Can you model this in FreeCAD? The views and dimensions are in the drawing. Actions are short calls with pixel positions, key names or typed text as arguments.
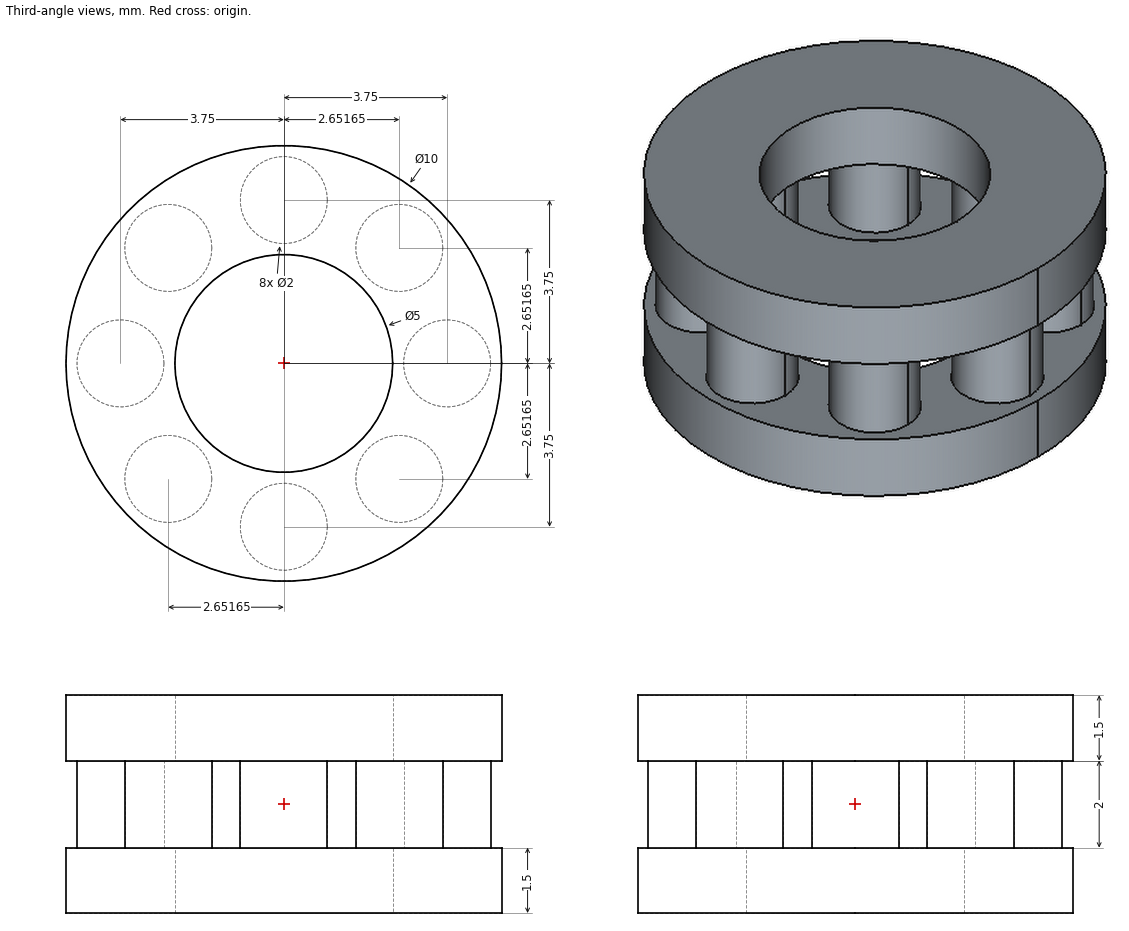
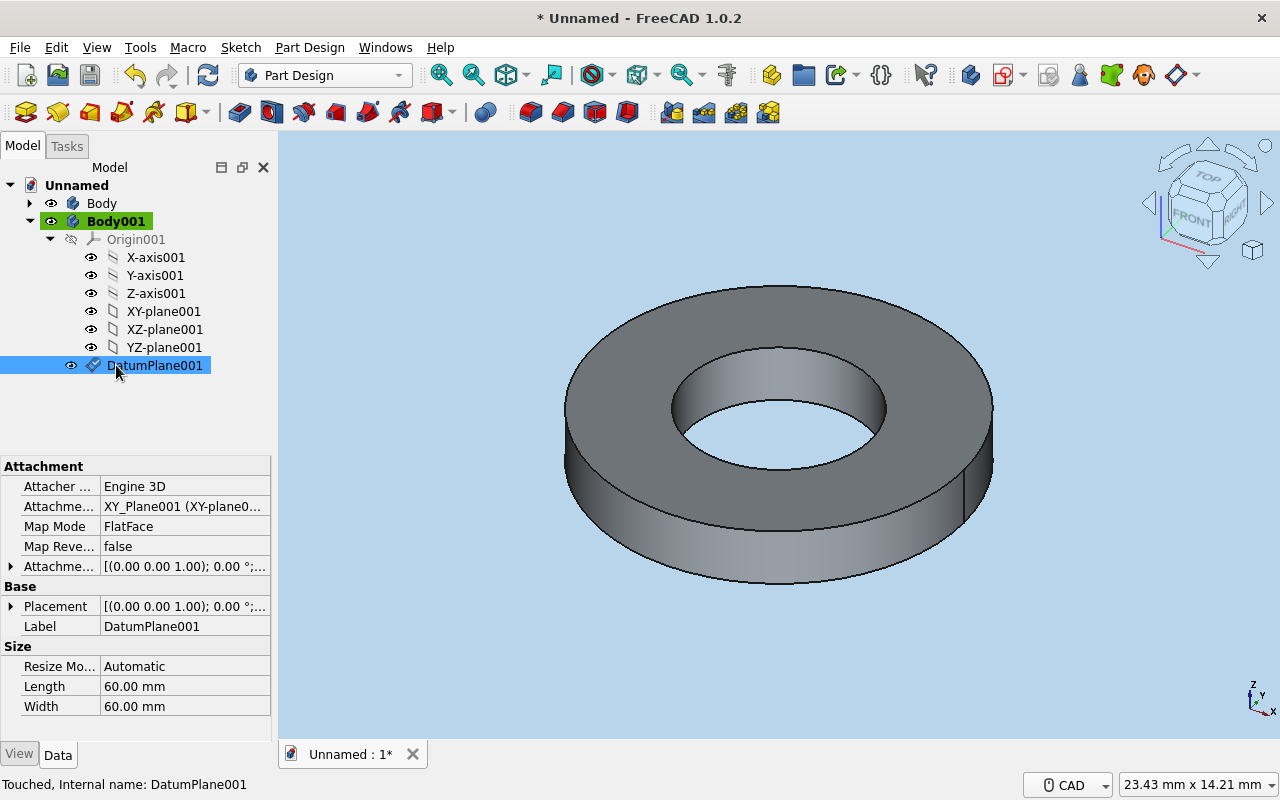
click(1004, 76)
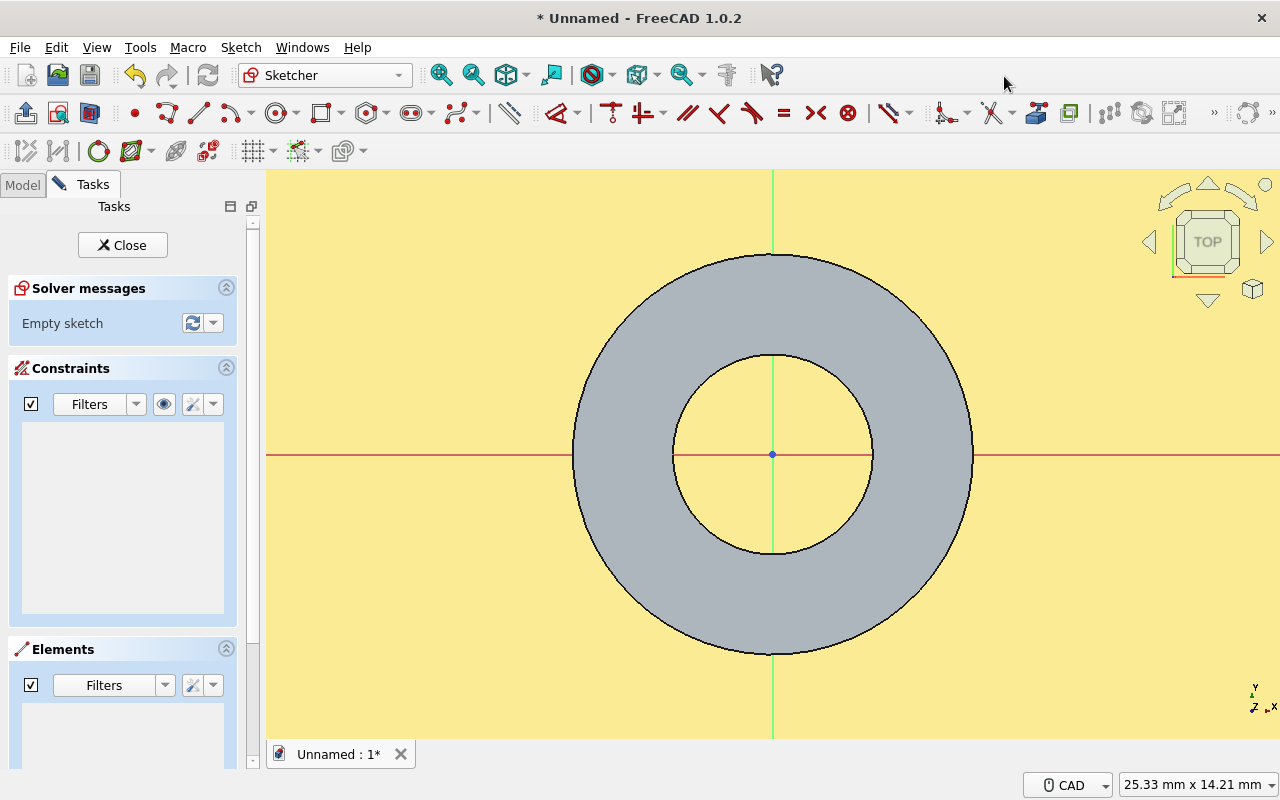
click(276, 114)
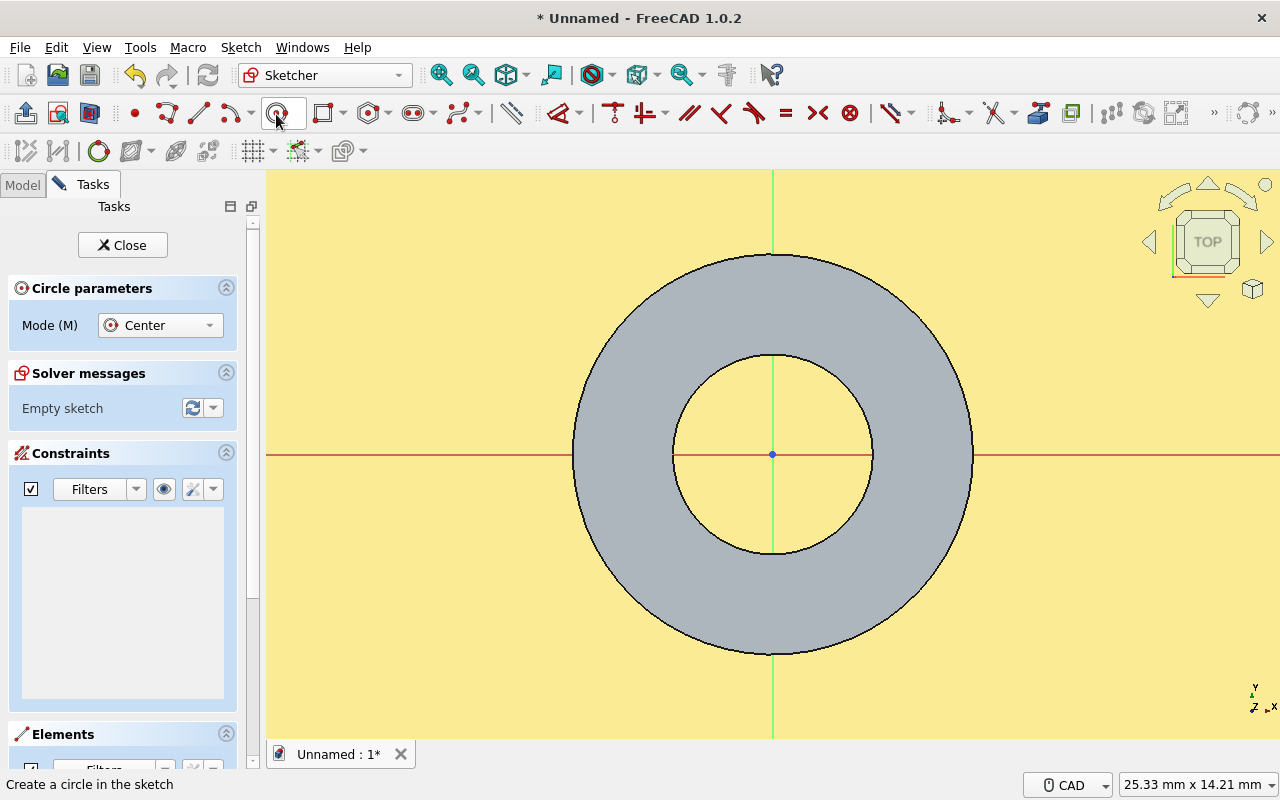
click(773, 454)
move(914, 313)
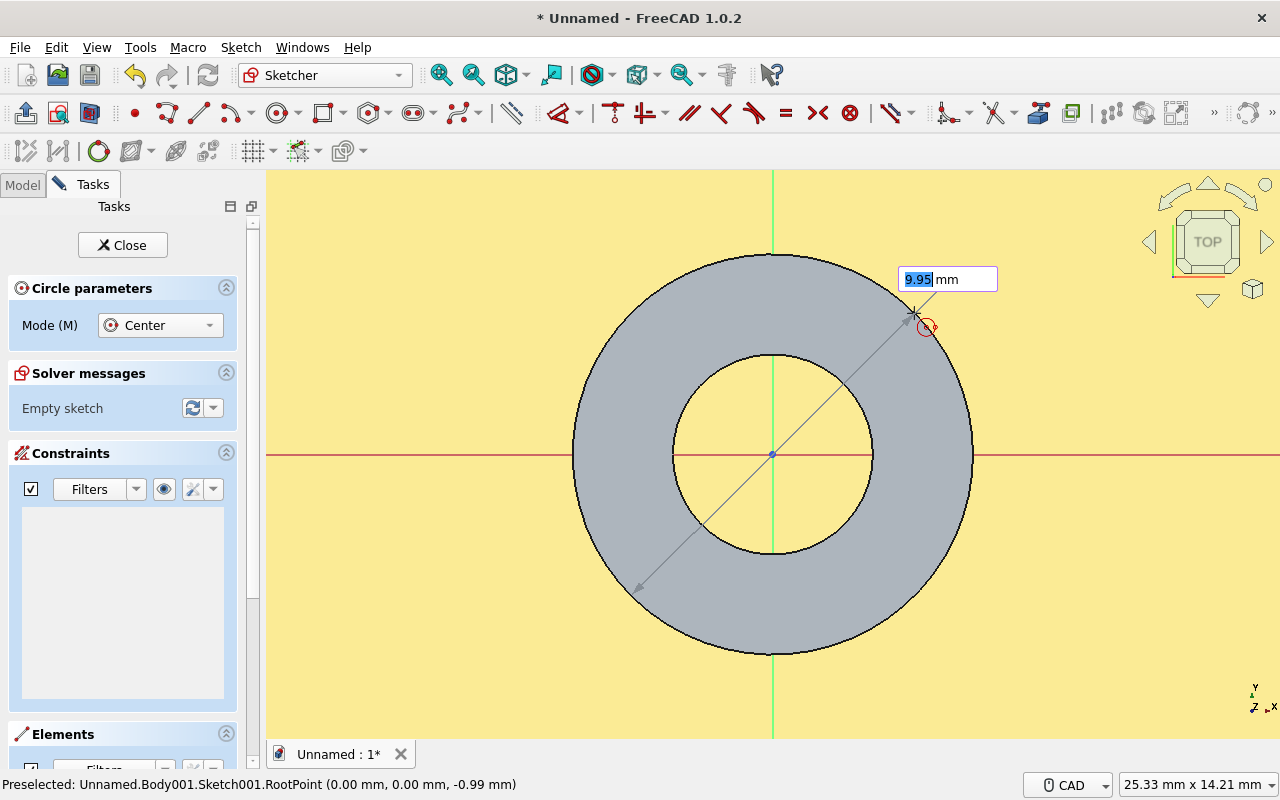
text(10)
key(Return)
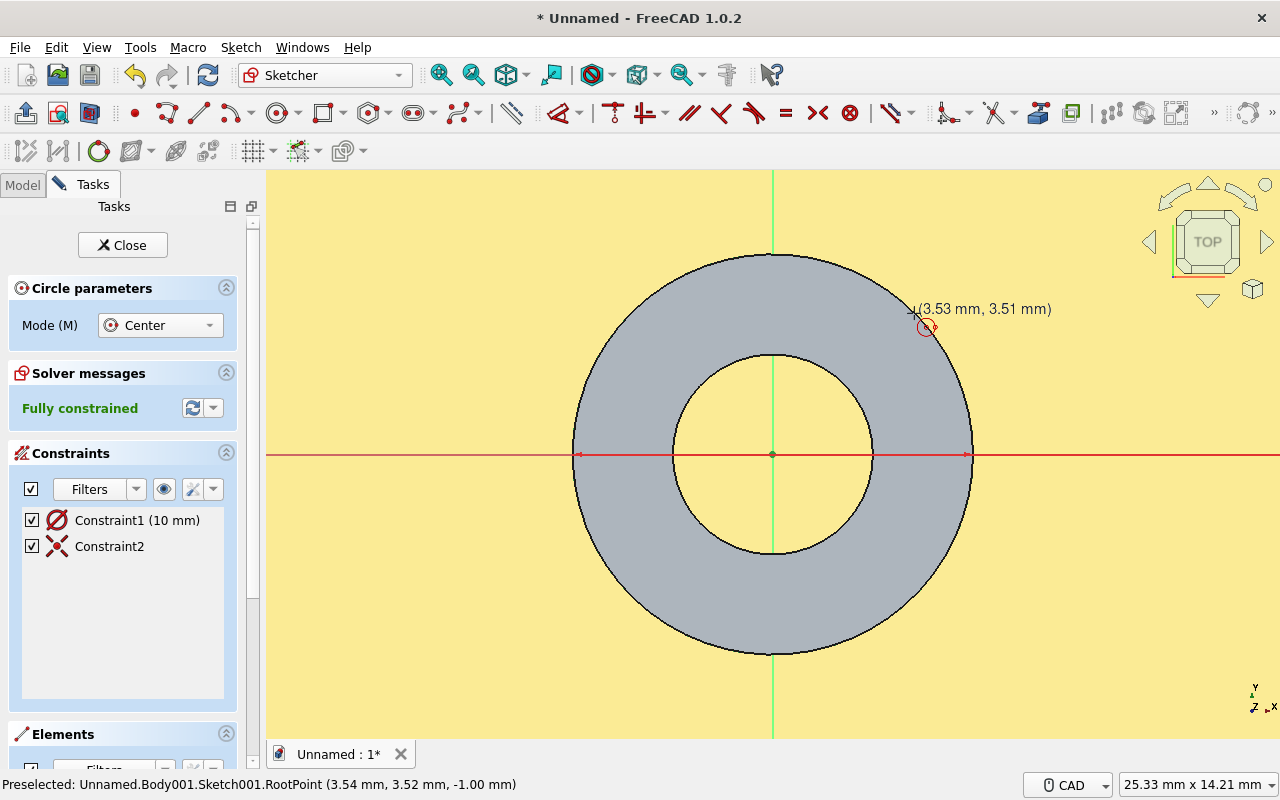
click(773, 454)
move(844, 384)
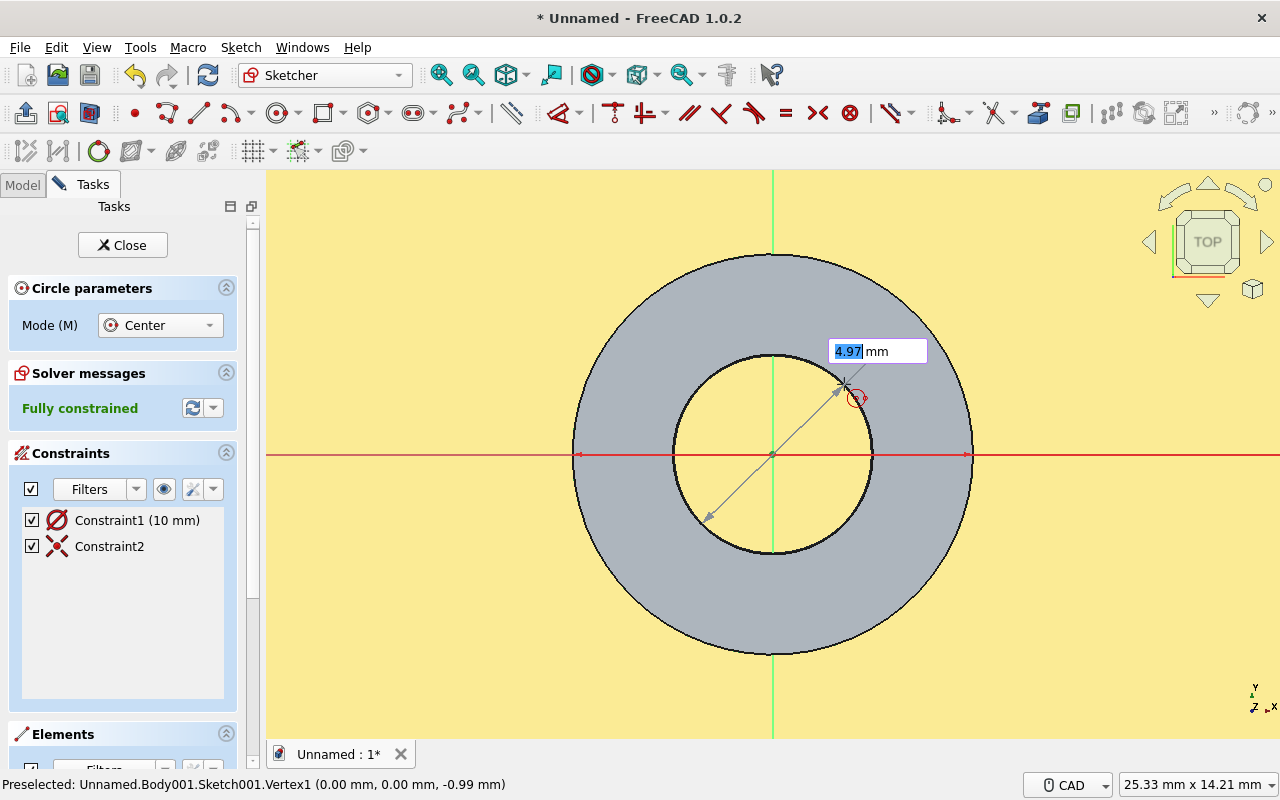
text(5)
key(Return)
key(Escape)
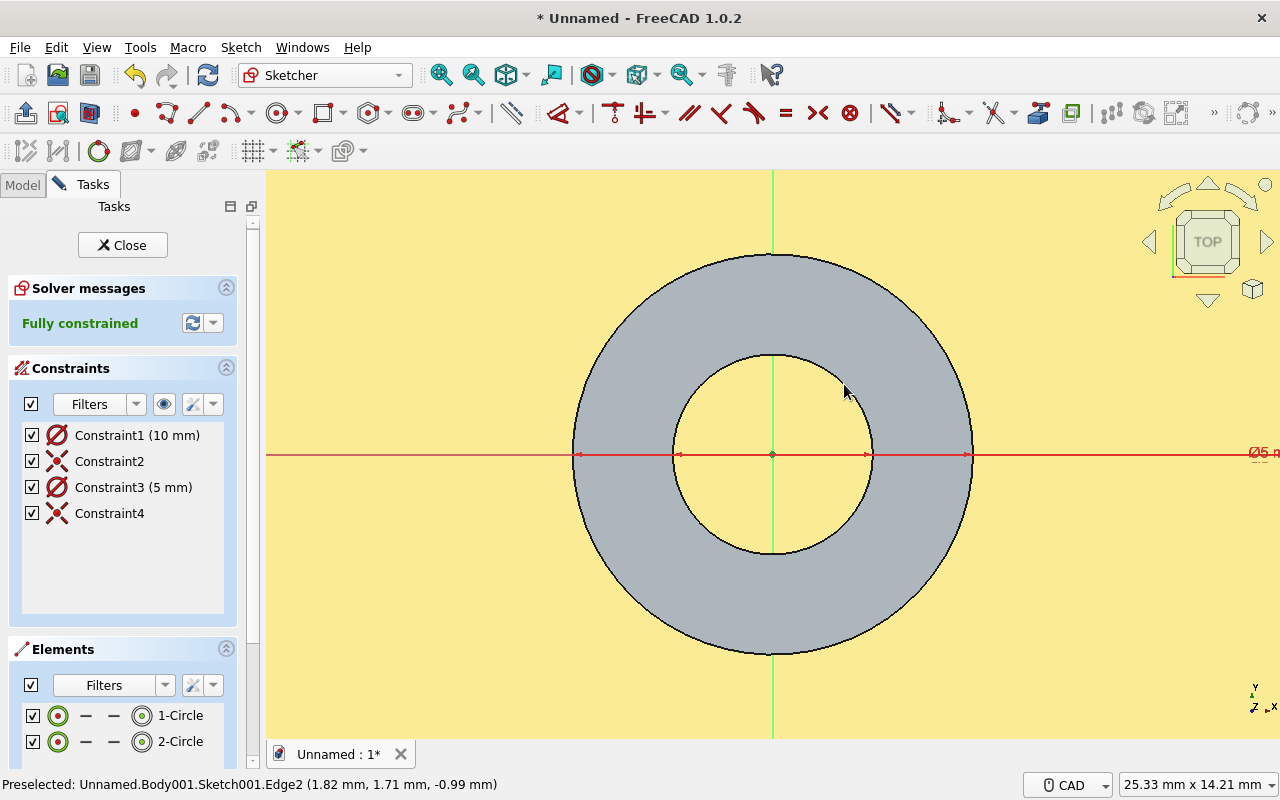
click(123, 245)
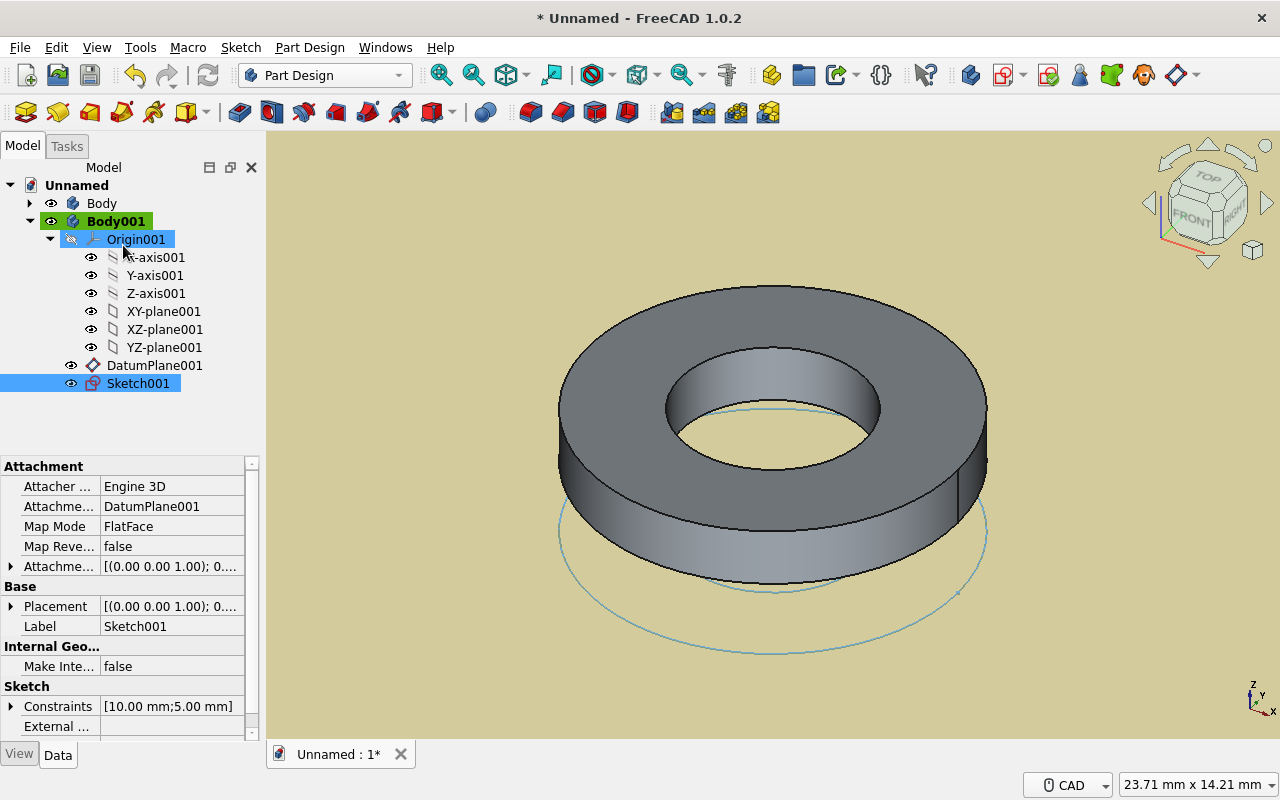
click(26, 112)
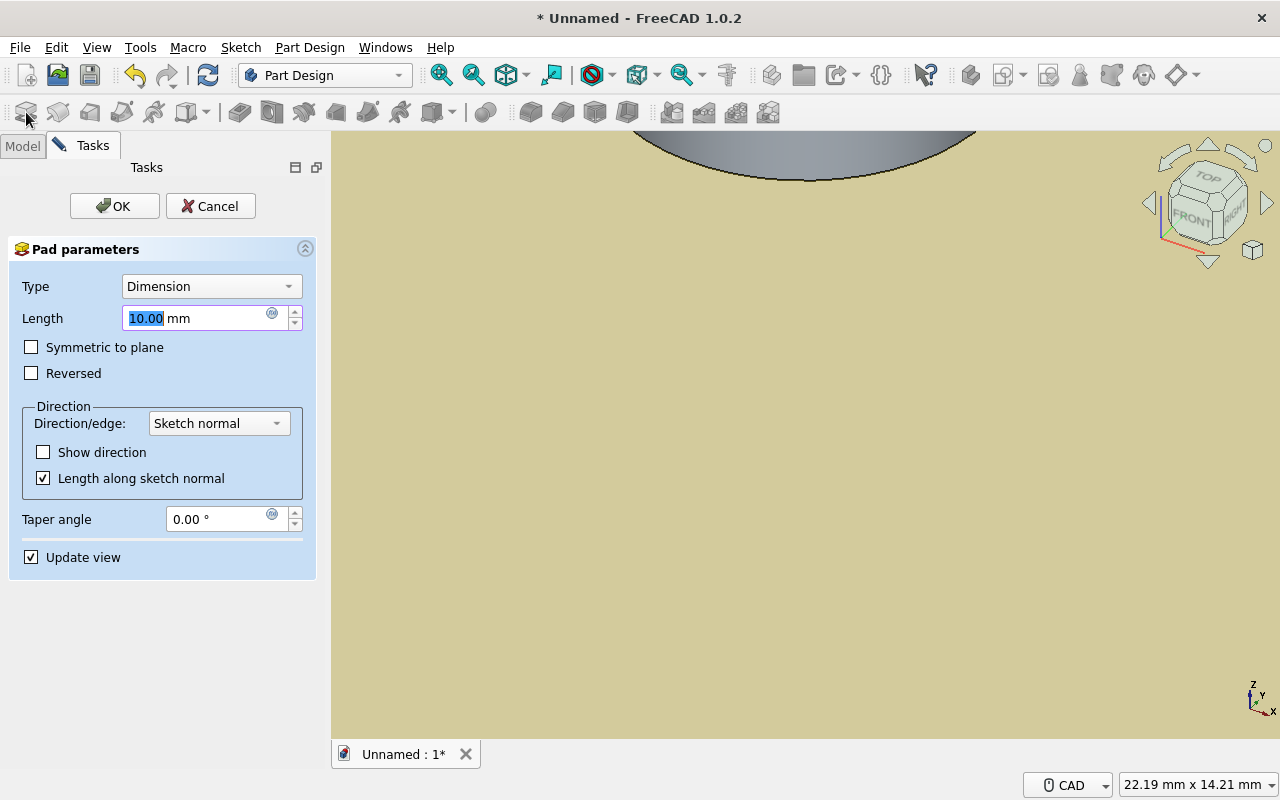
text(1.5)
key(Tab)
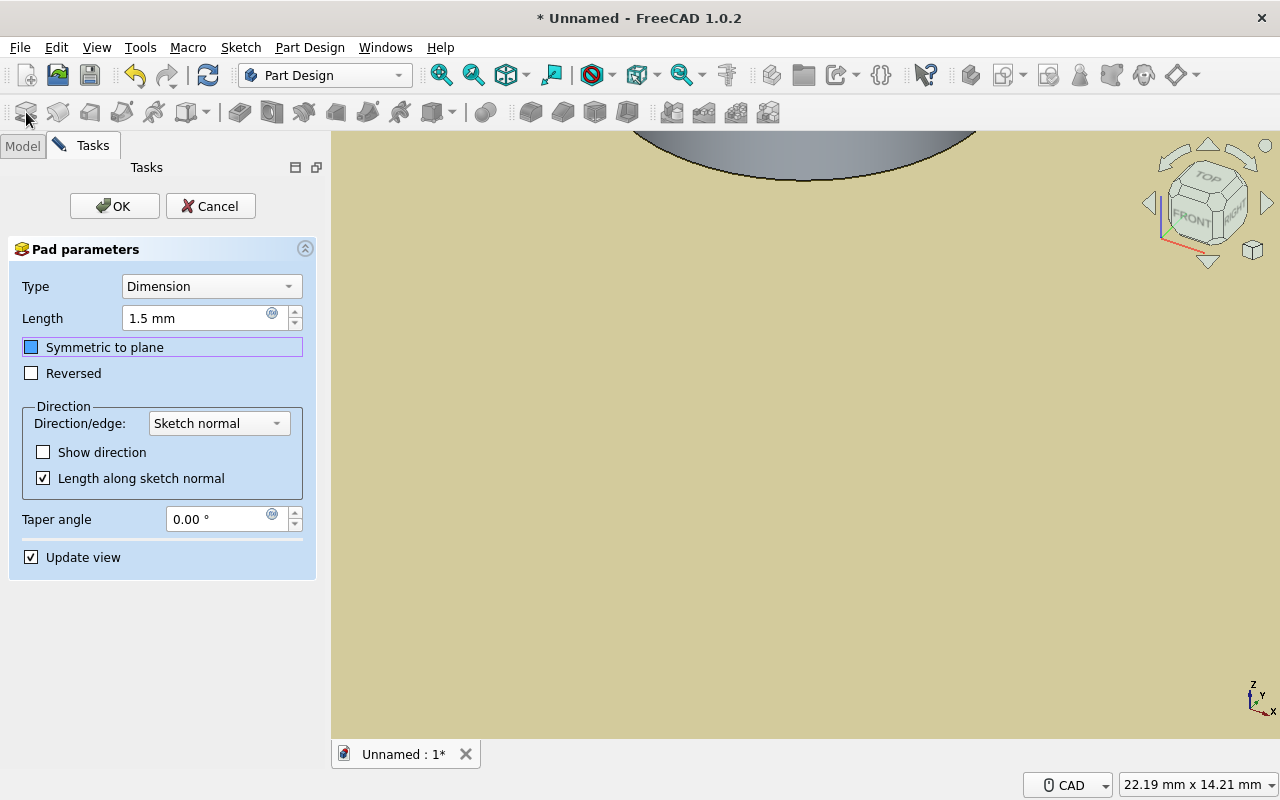
click(30, 373)